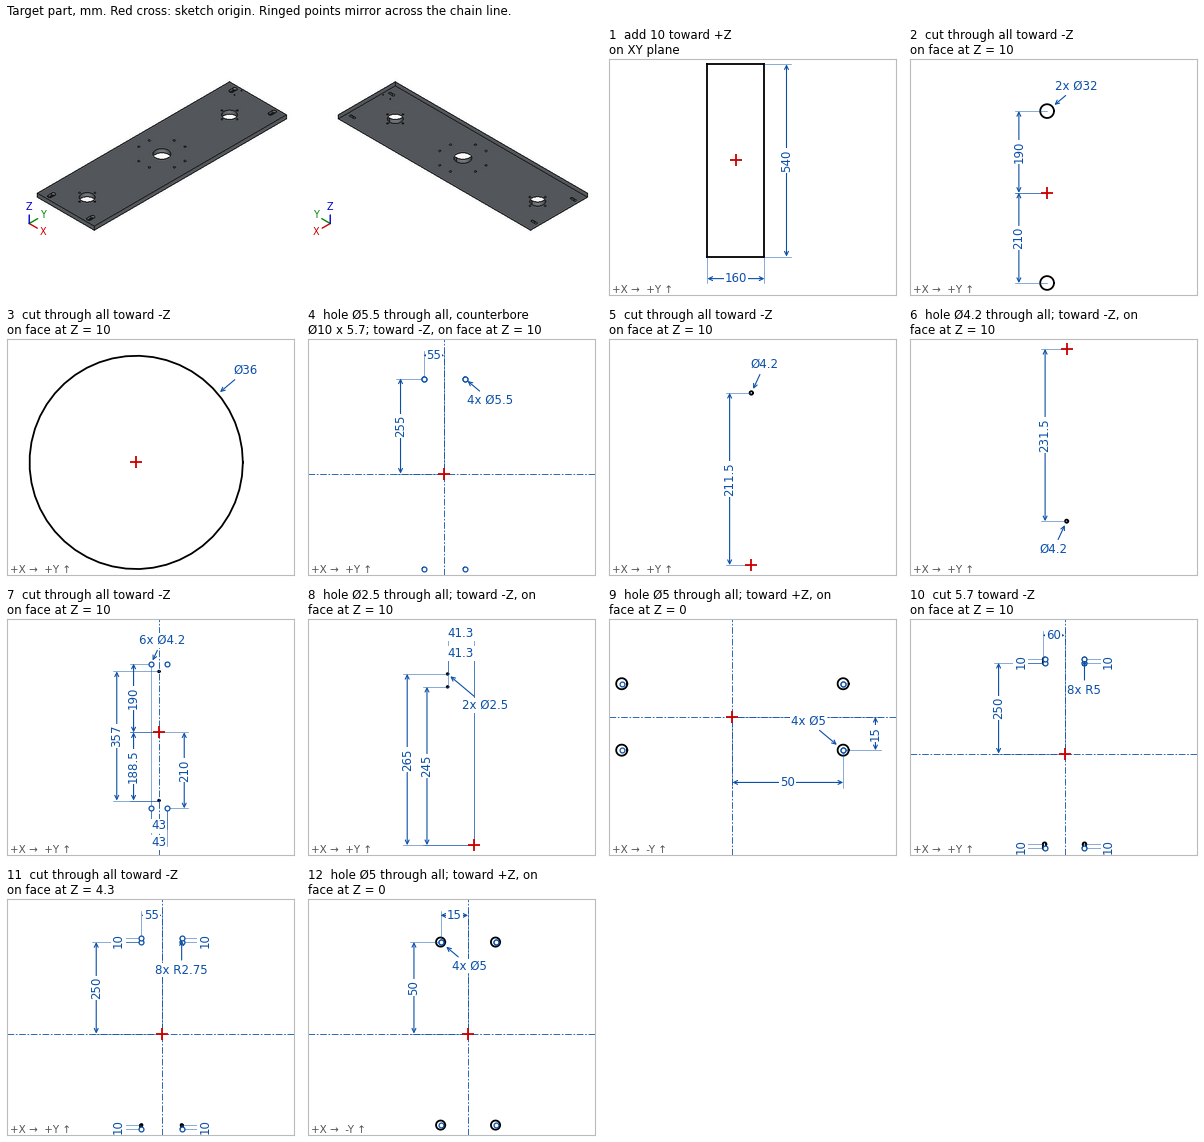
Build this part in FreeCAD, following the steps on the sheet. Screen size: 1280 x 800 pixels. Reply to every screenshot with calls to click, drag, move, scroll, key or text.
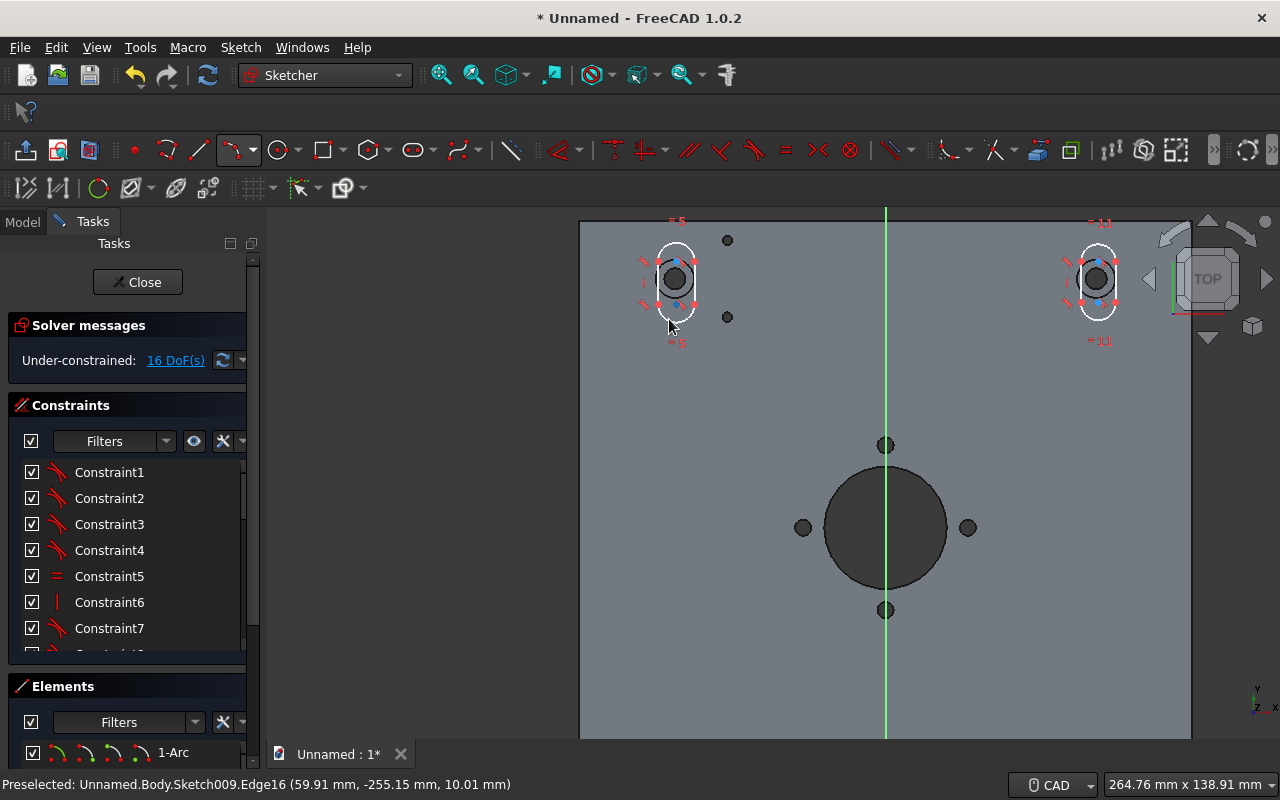
click(666, 319)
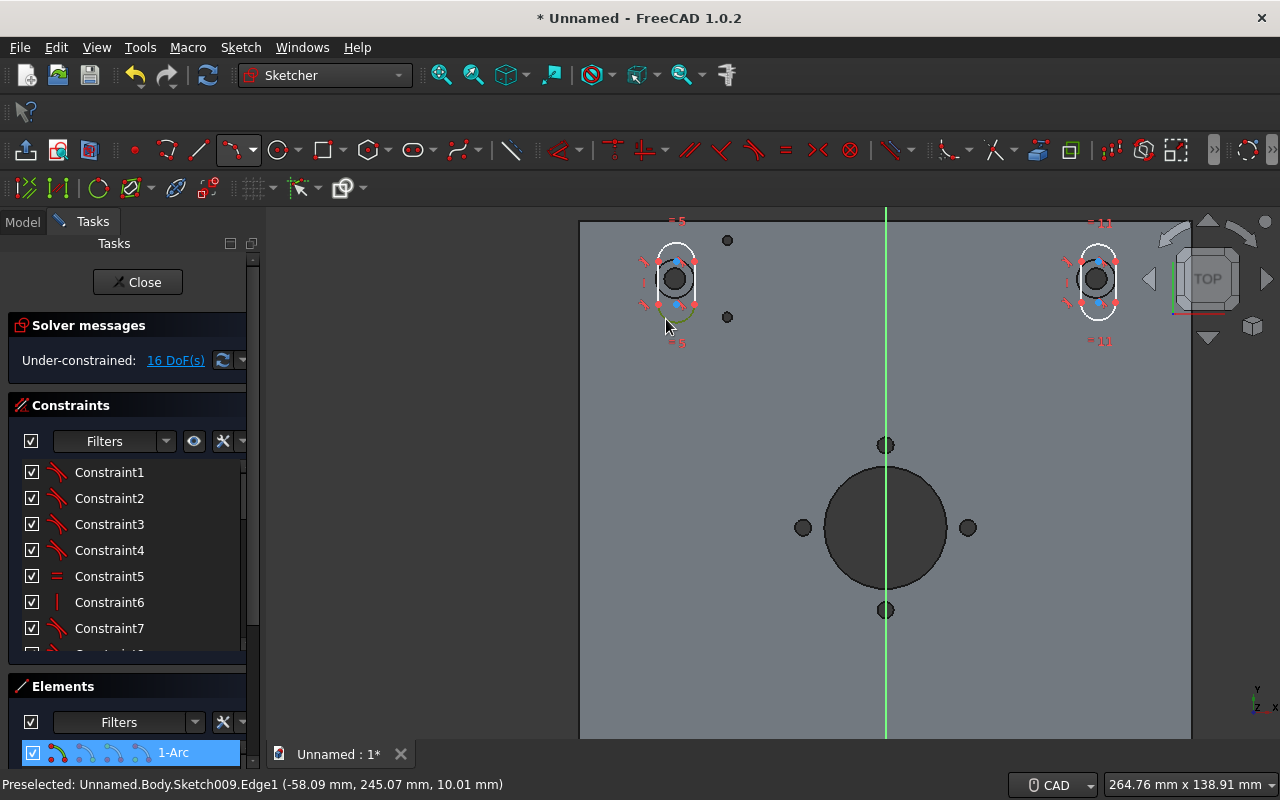
click(1088, 317)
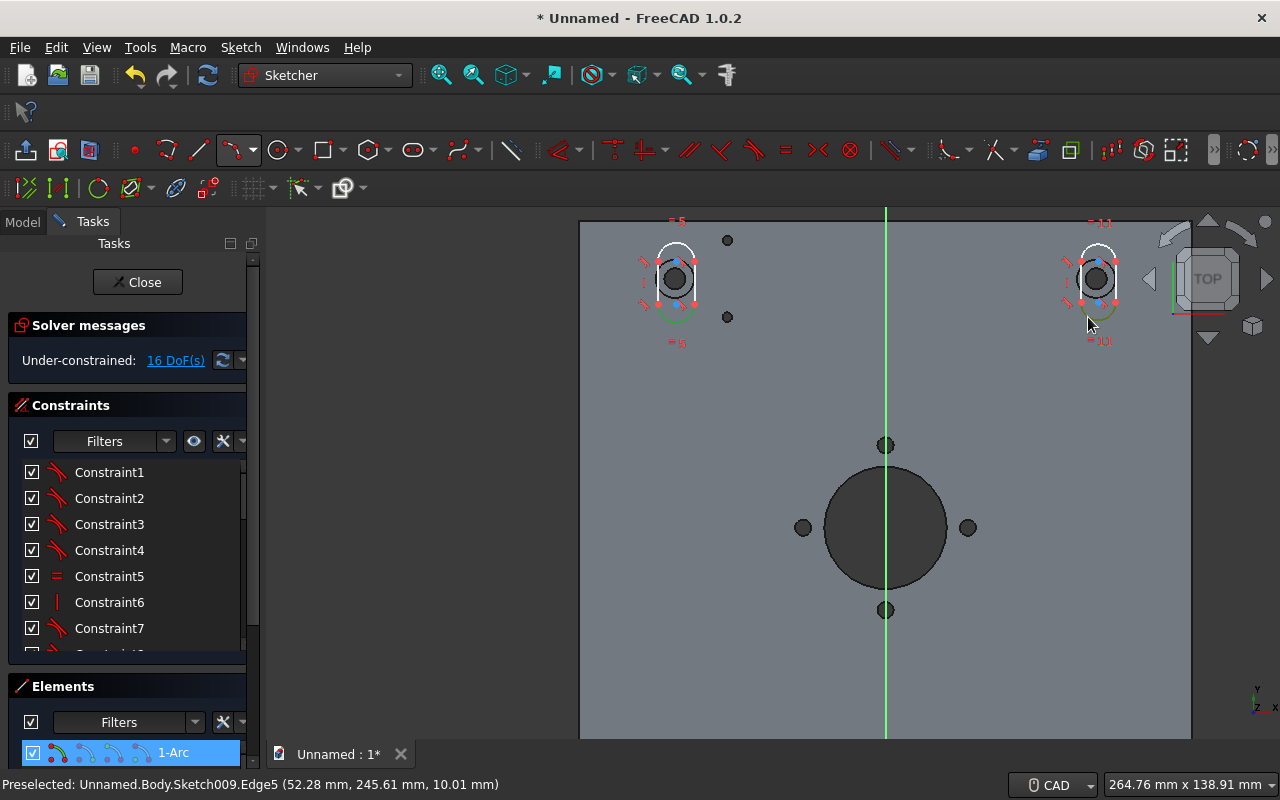
scroll(669, 318, down, 9)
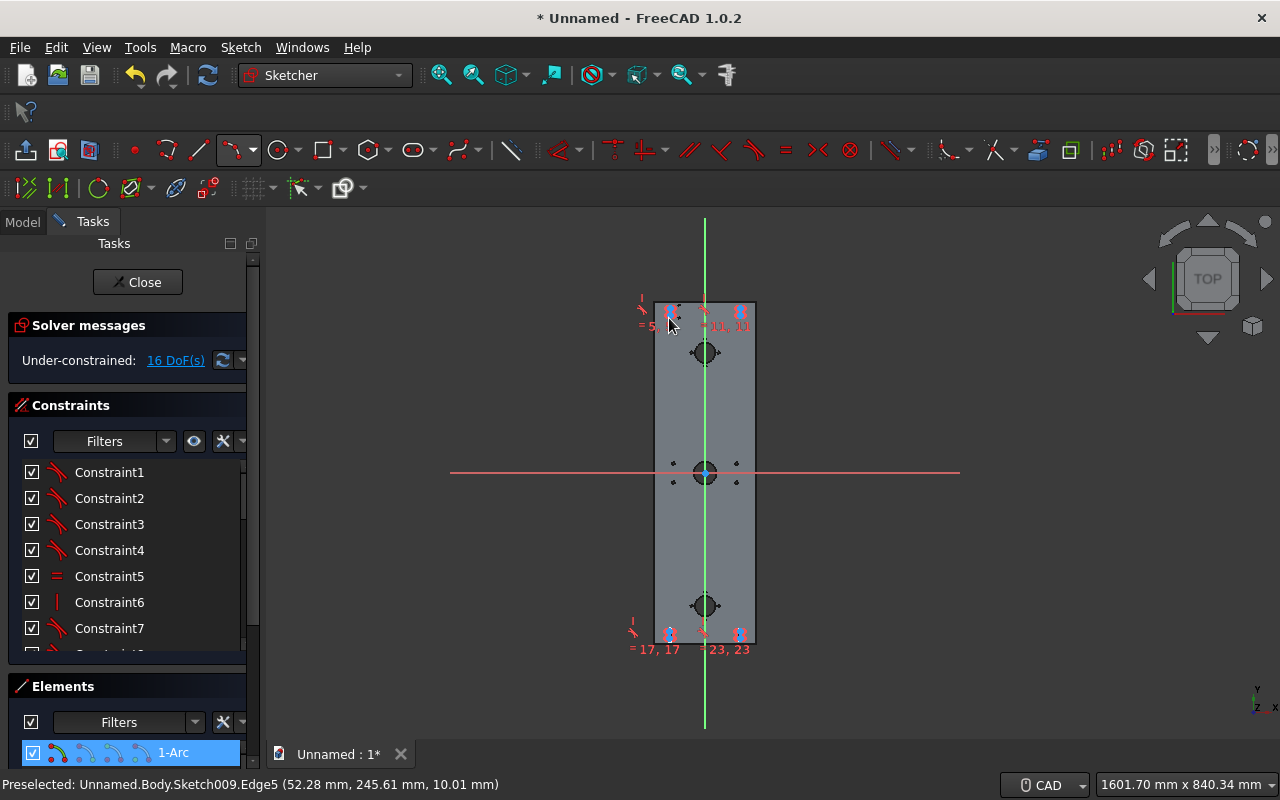
scroll(668, 641, up, 8)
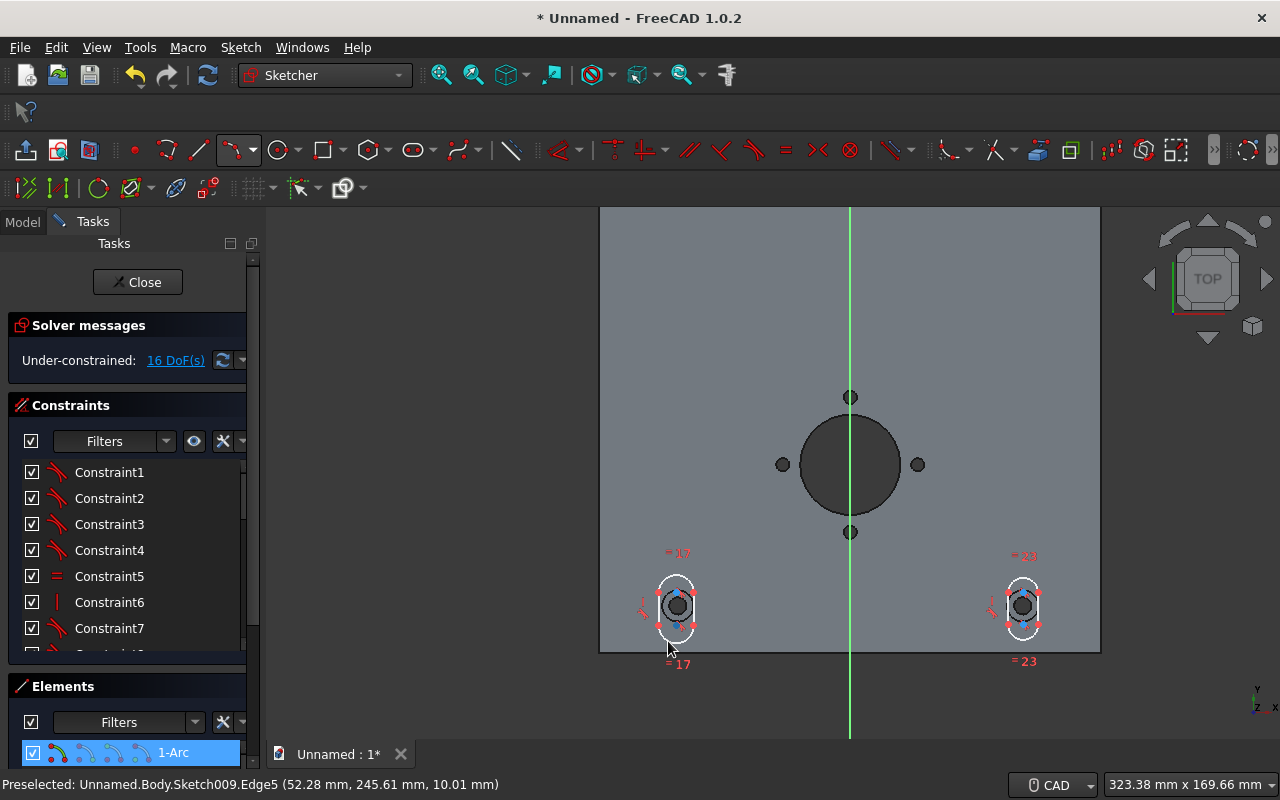
click(666, 640)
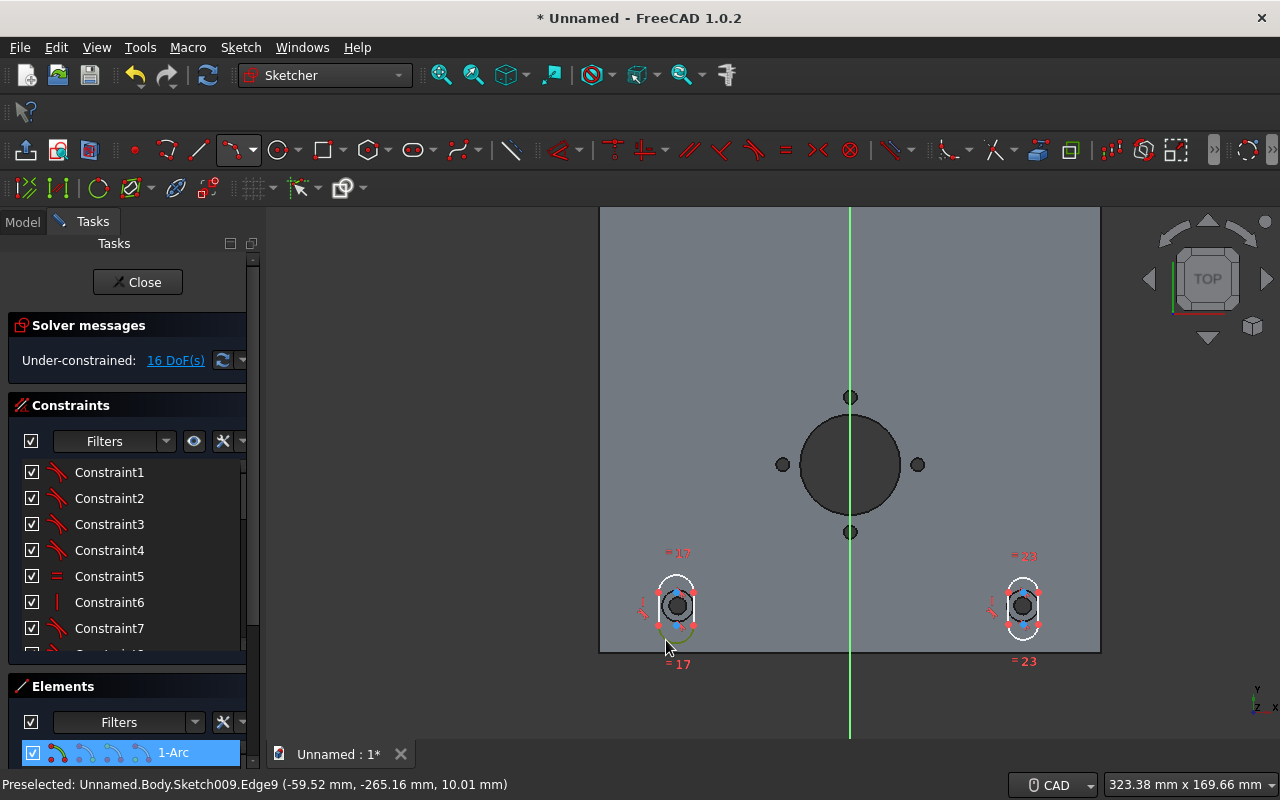
click(1014, 637)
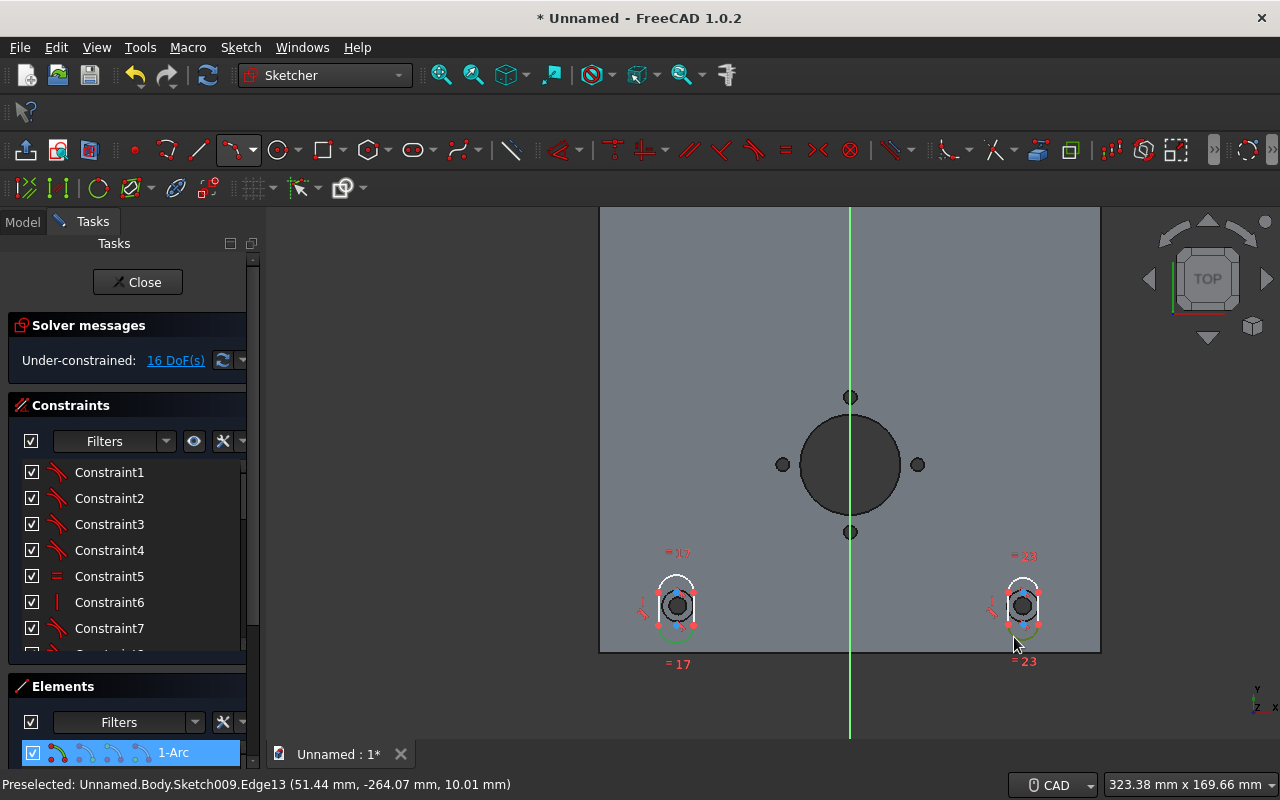
click(786, 150)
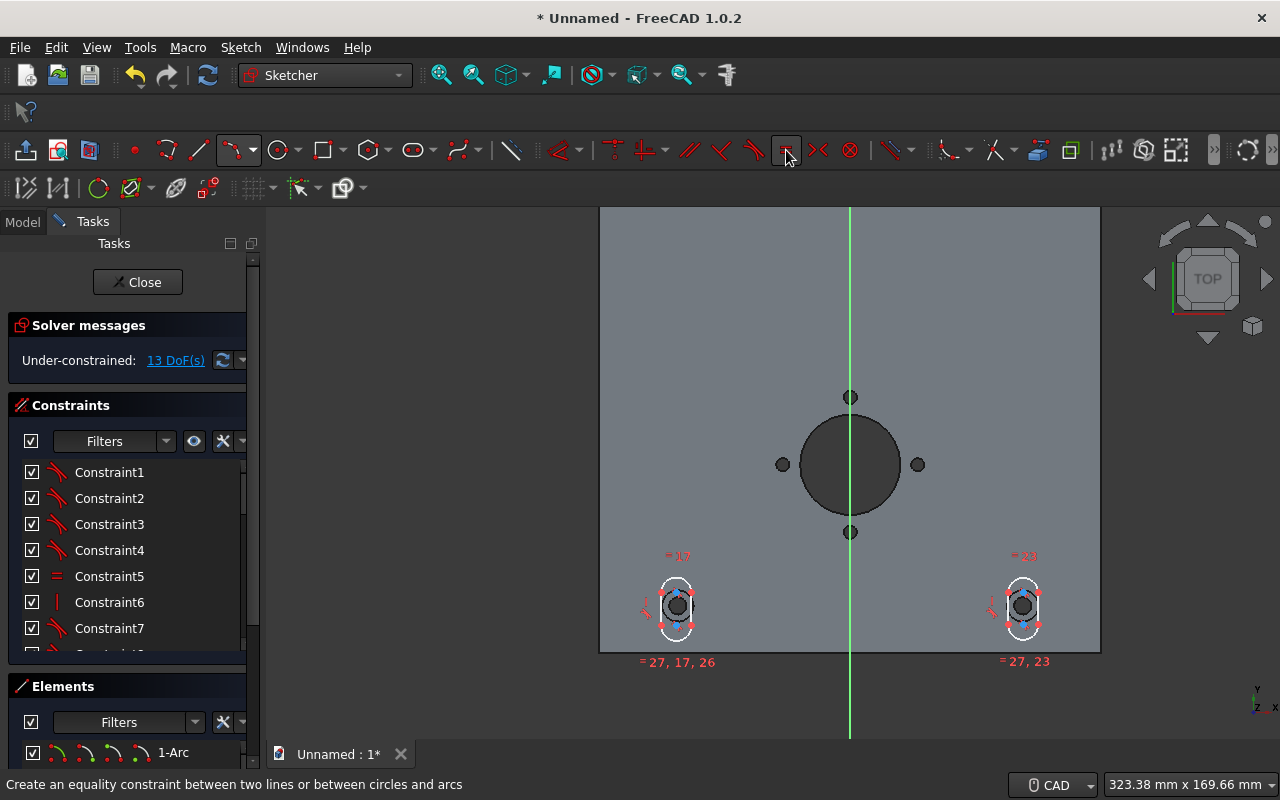
scroll(668, 642, down, 8)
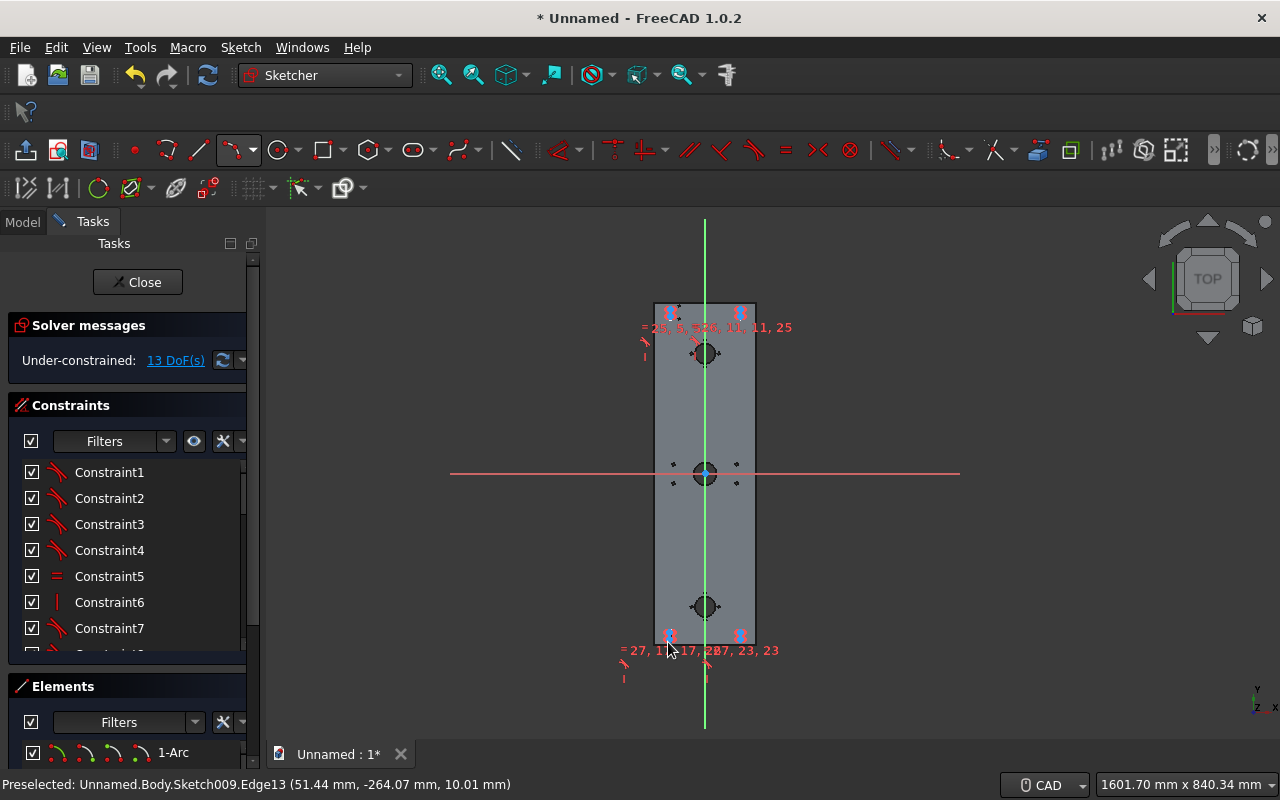
scroll(670, 317, up, 7)